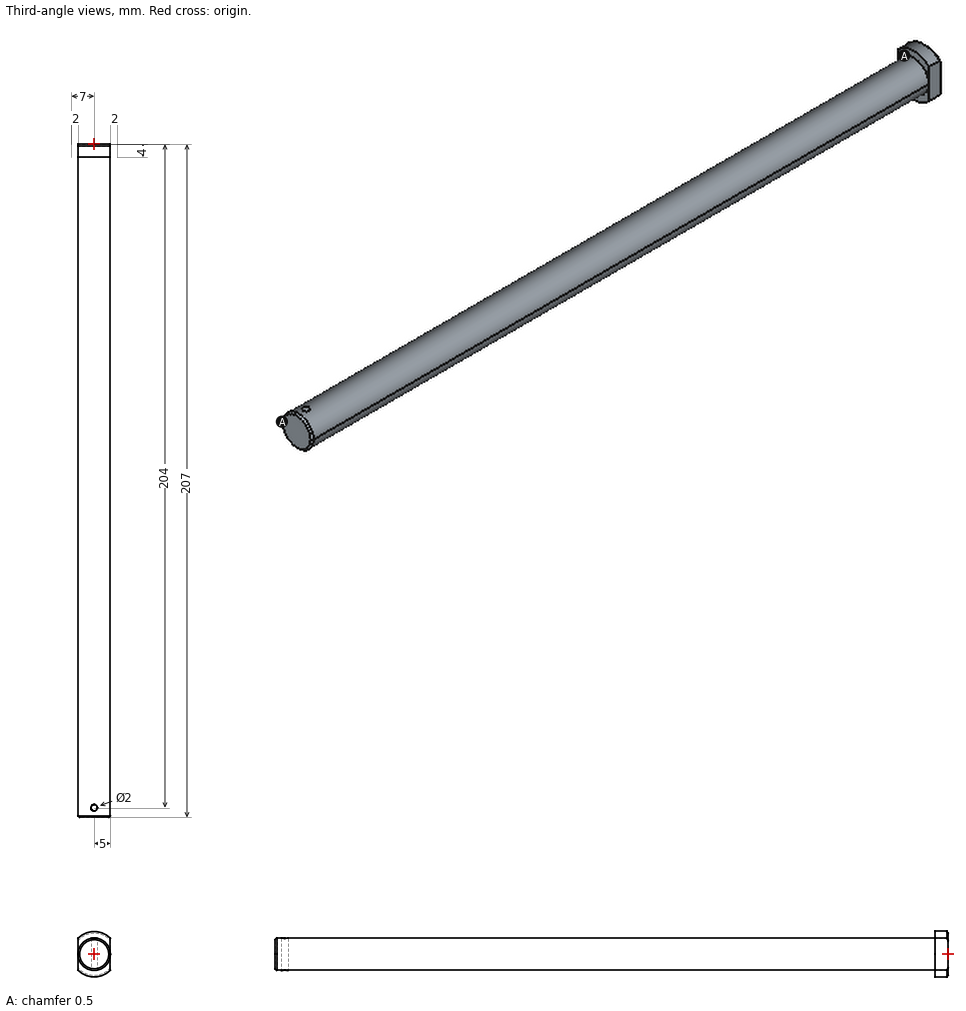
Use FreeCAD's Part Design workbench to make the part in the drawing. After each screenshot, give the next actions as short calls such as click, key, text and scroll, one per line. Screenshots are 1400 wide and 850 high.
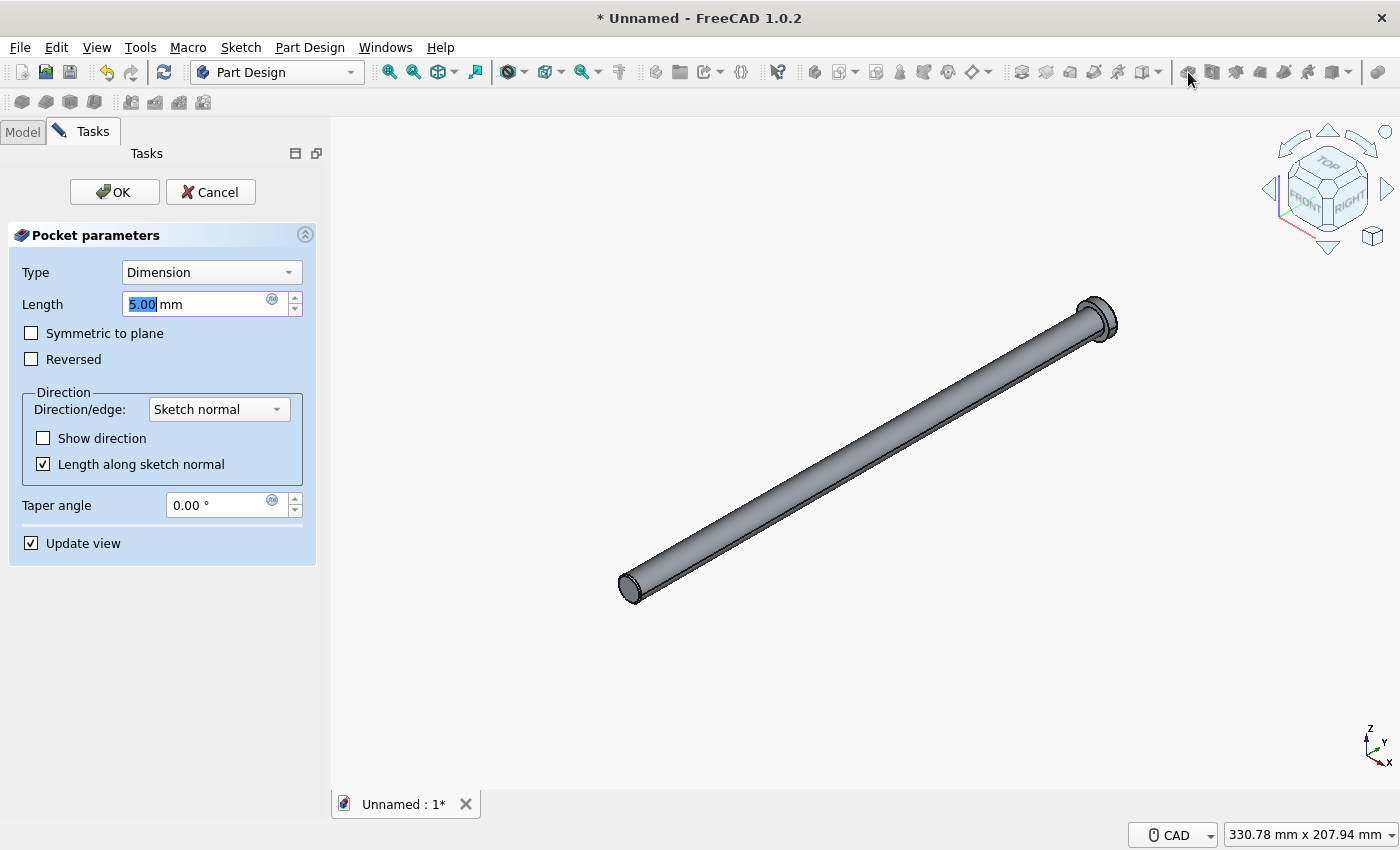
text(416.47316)
key(Tab)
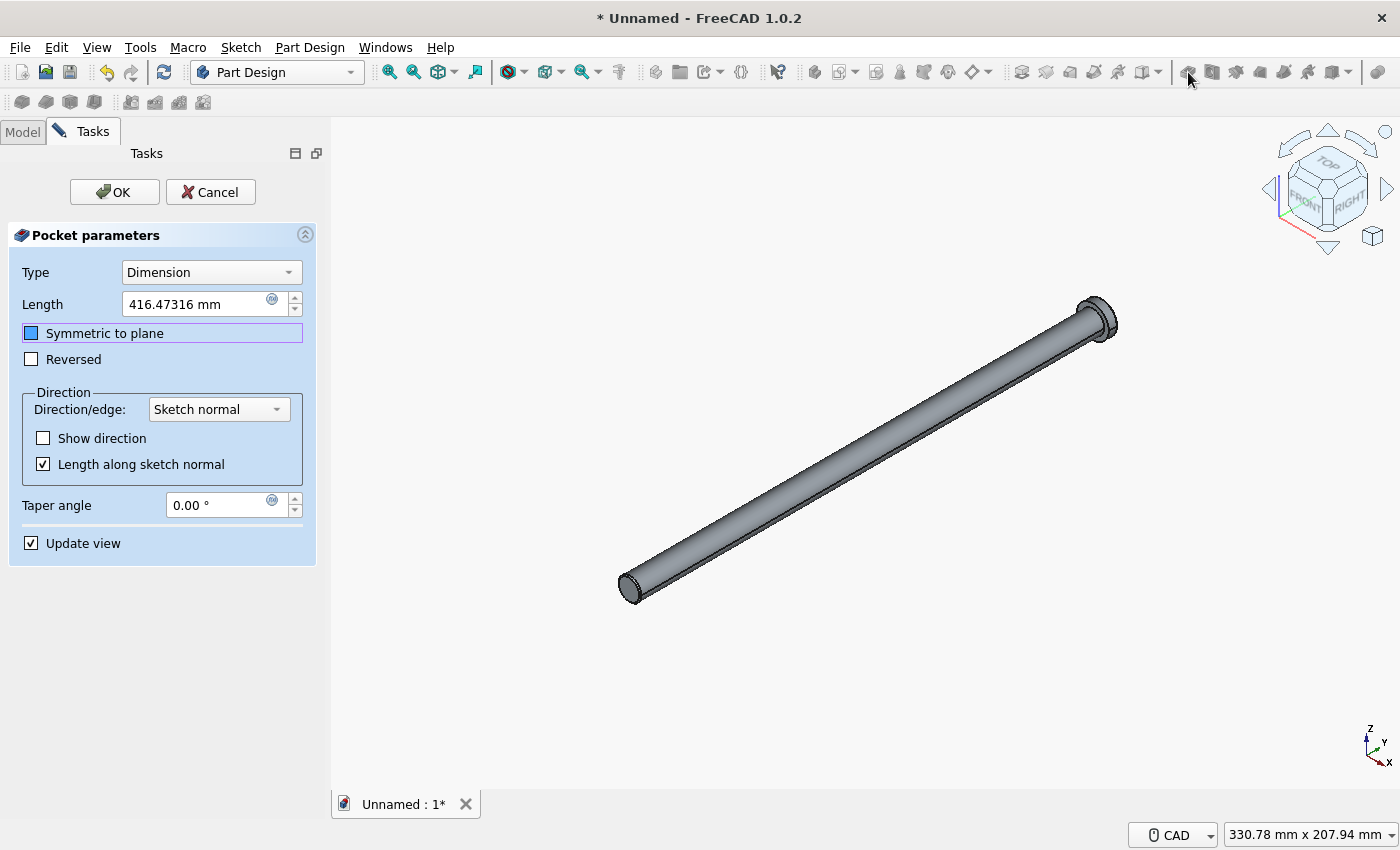
click(30, 333)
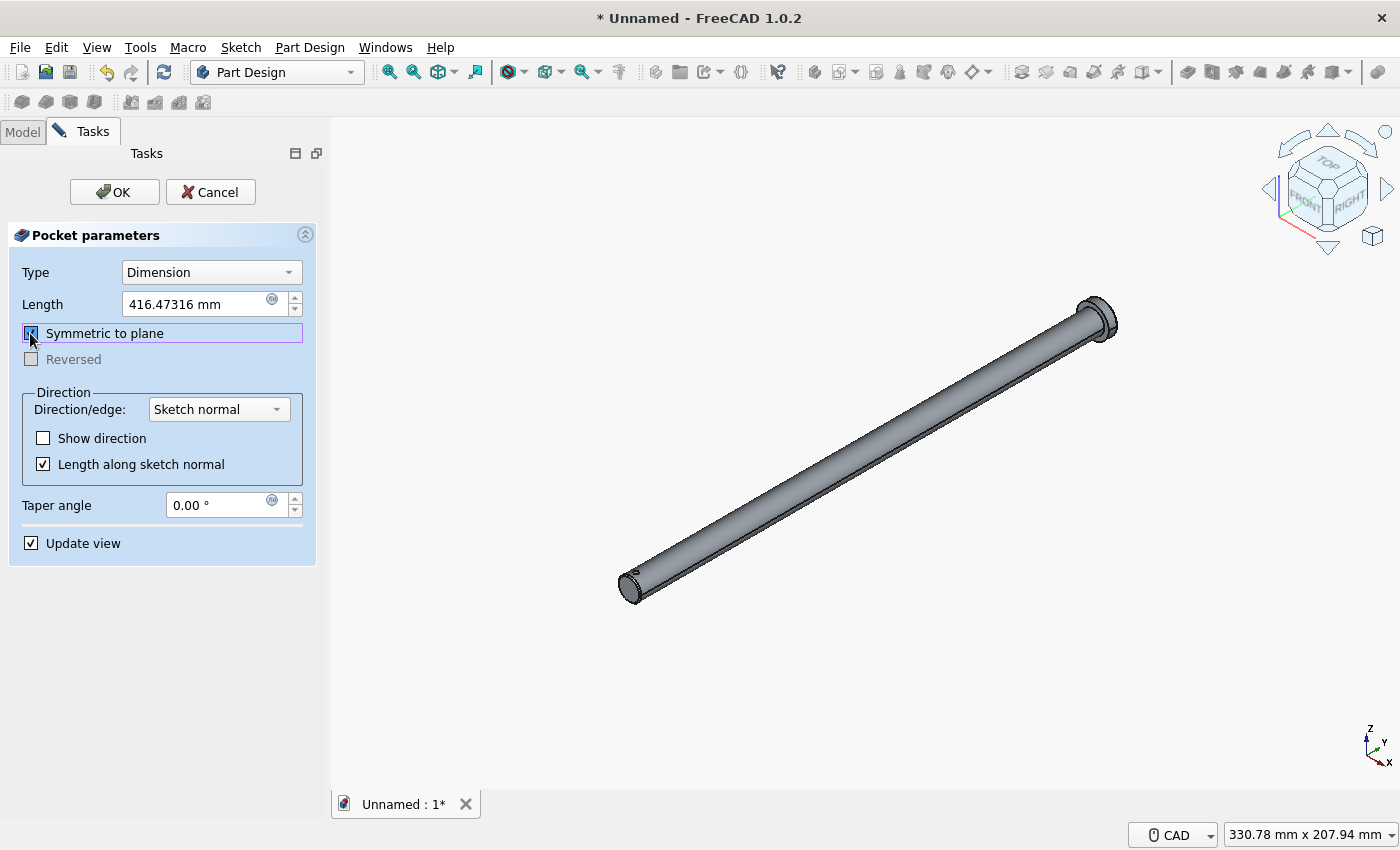
click(115, 192)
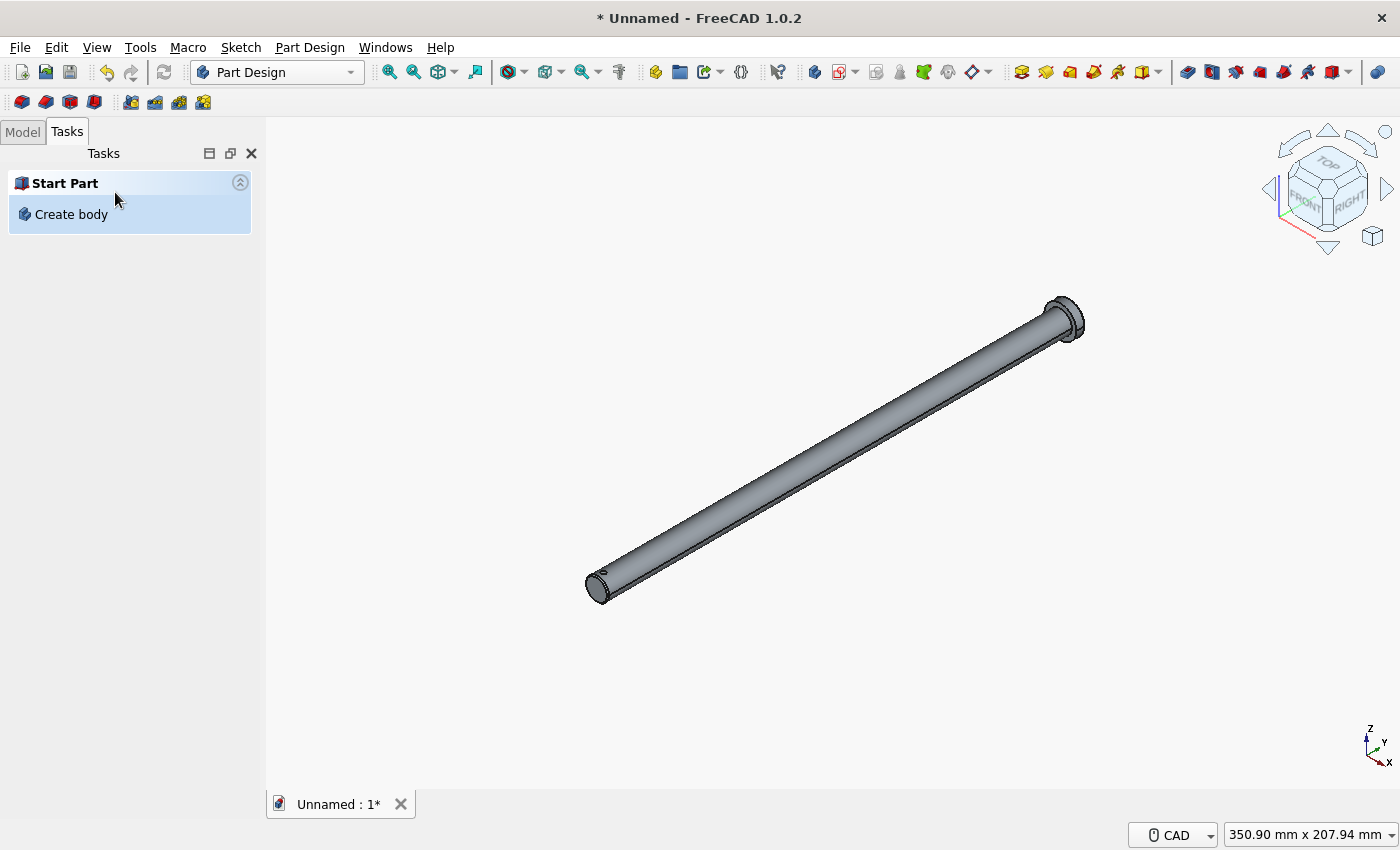
click(840, 72)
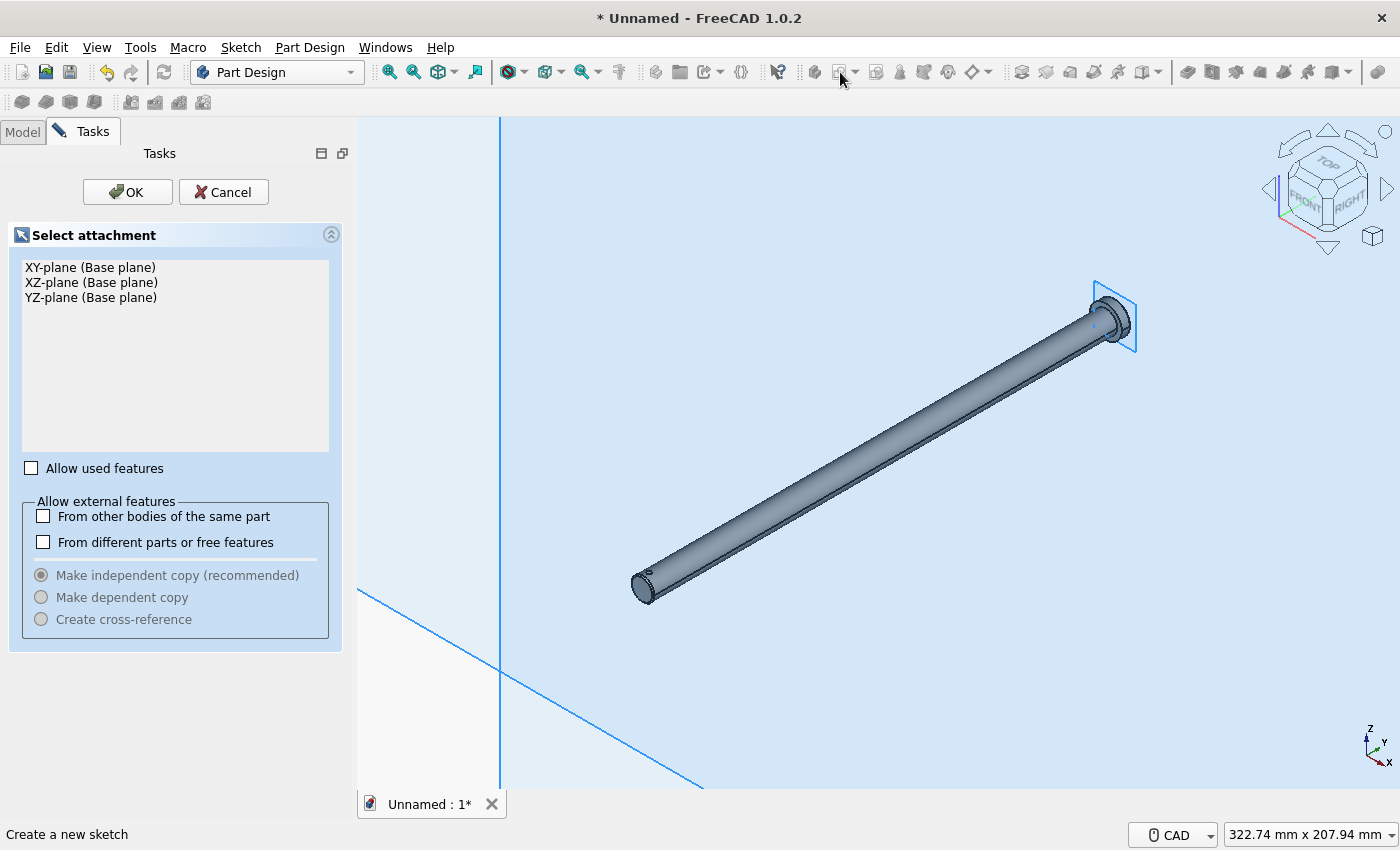
click(82, 268)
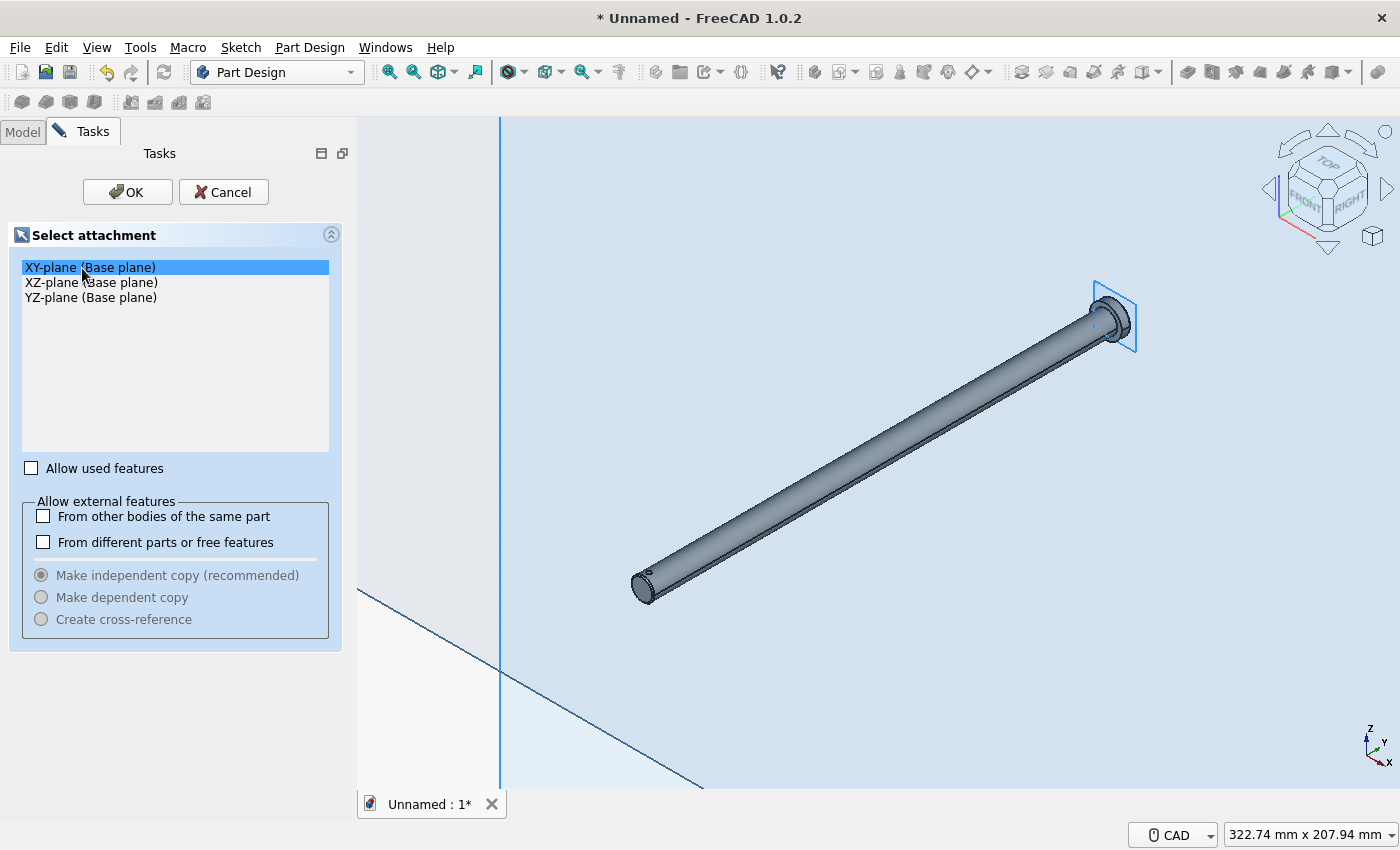
click(128, 192)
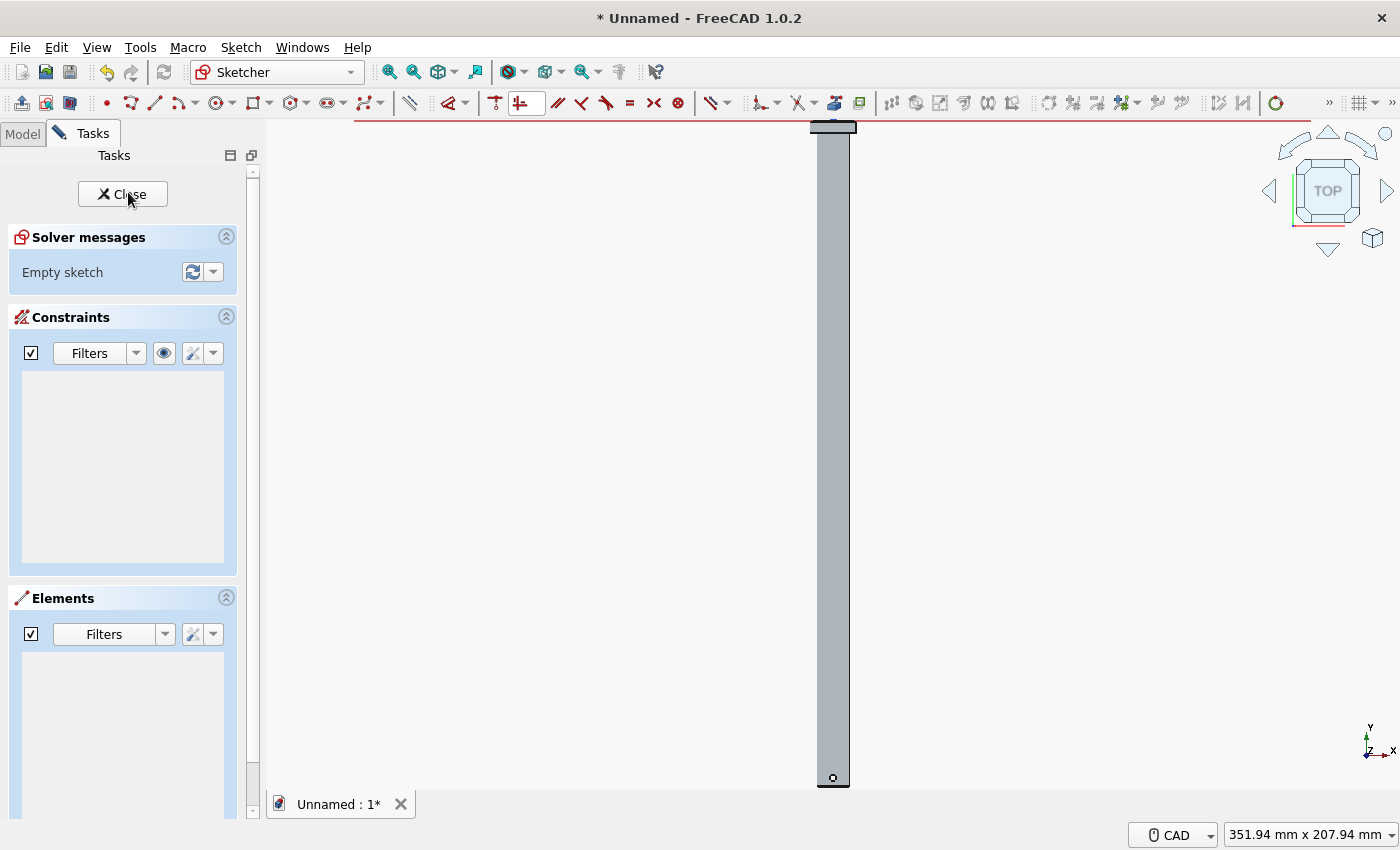
click(70, 104)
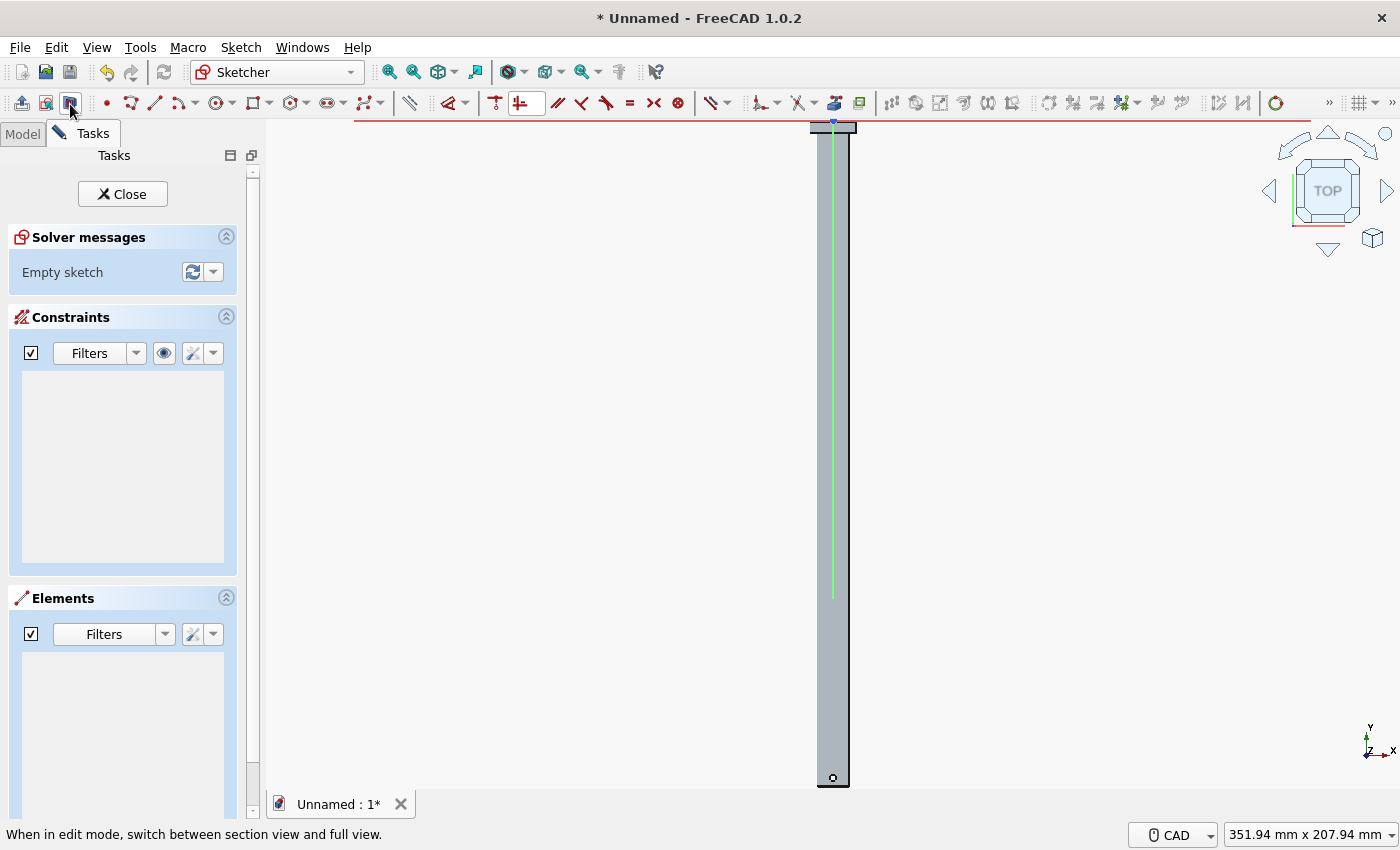
scroll(764, 454, down, 5)